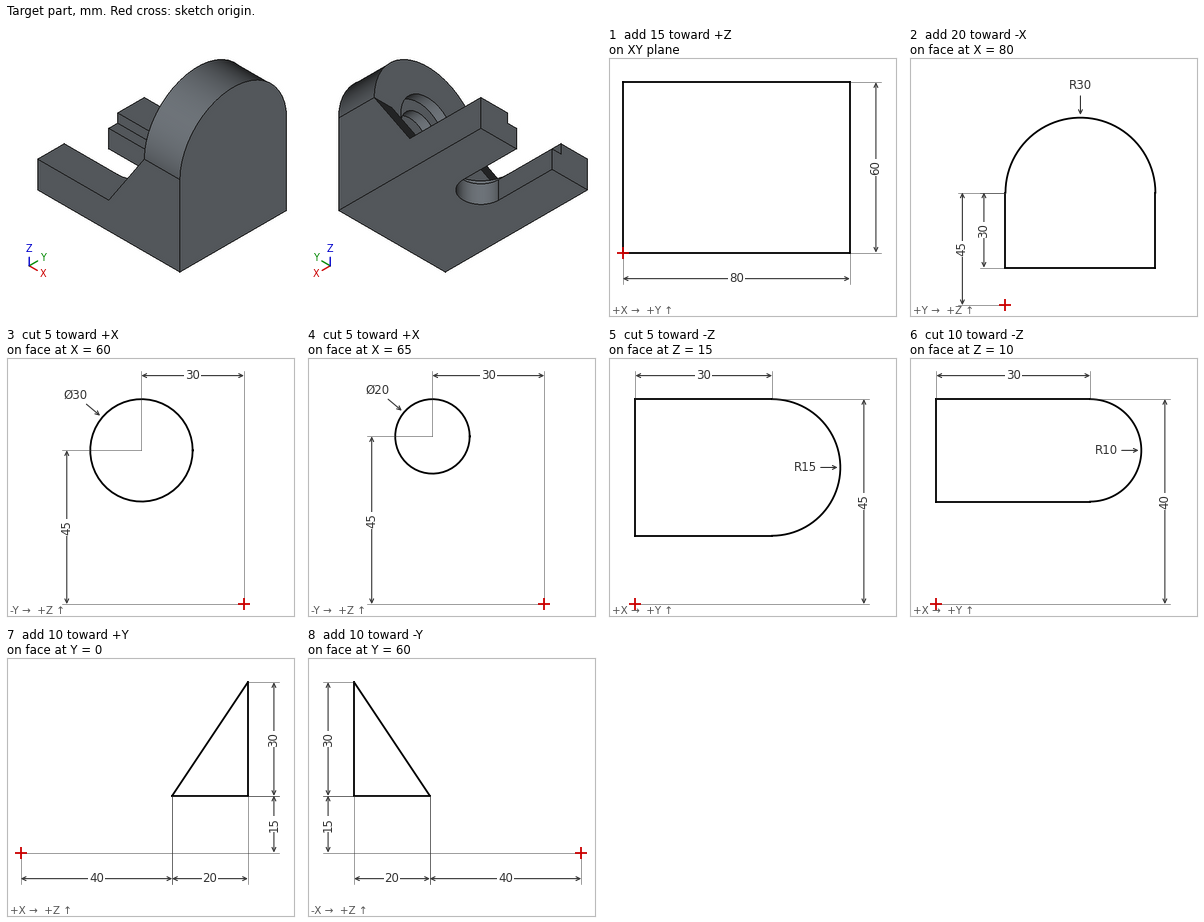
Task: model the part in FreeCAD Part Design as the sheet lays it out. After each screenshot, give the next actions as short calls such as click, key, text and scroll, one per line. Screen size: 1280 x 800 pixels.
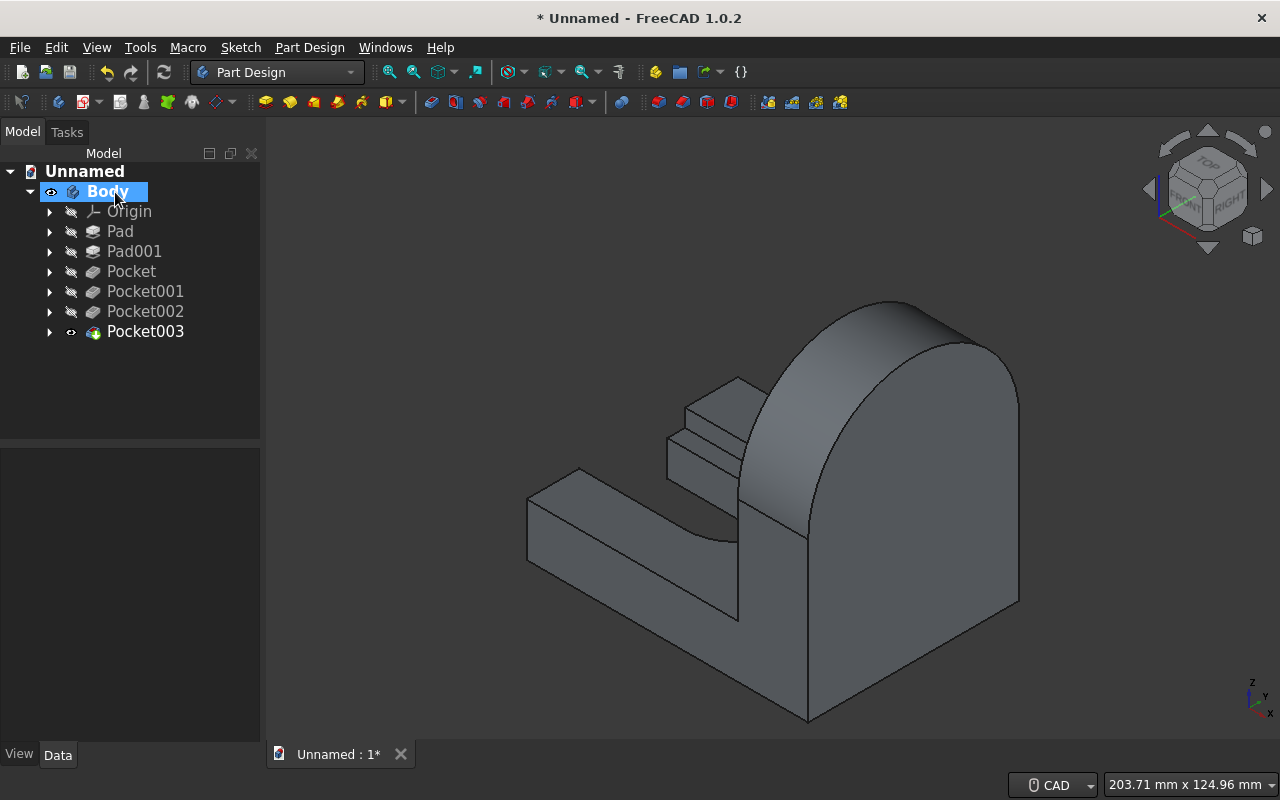
click(748, 647)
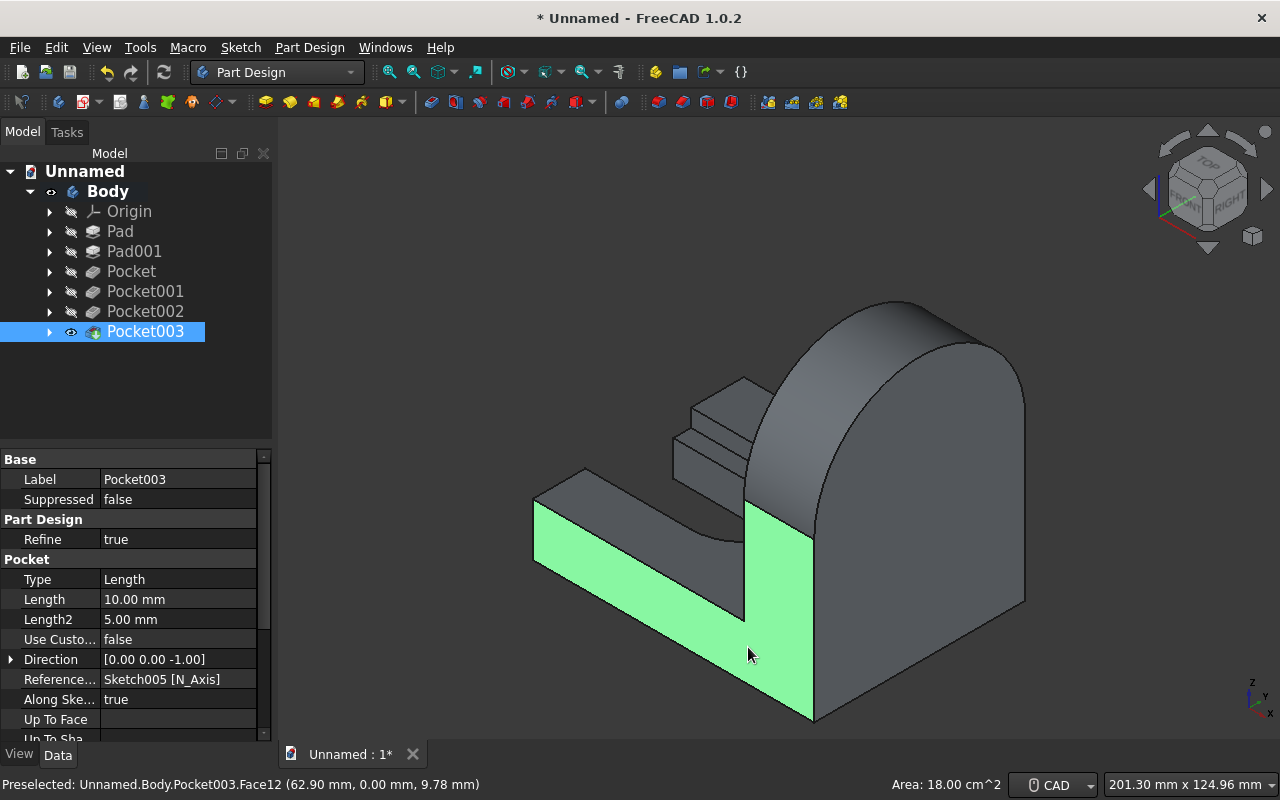
click(84, 102)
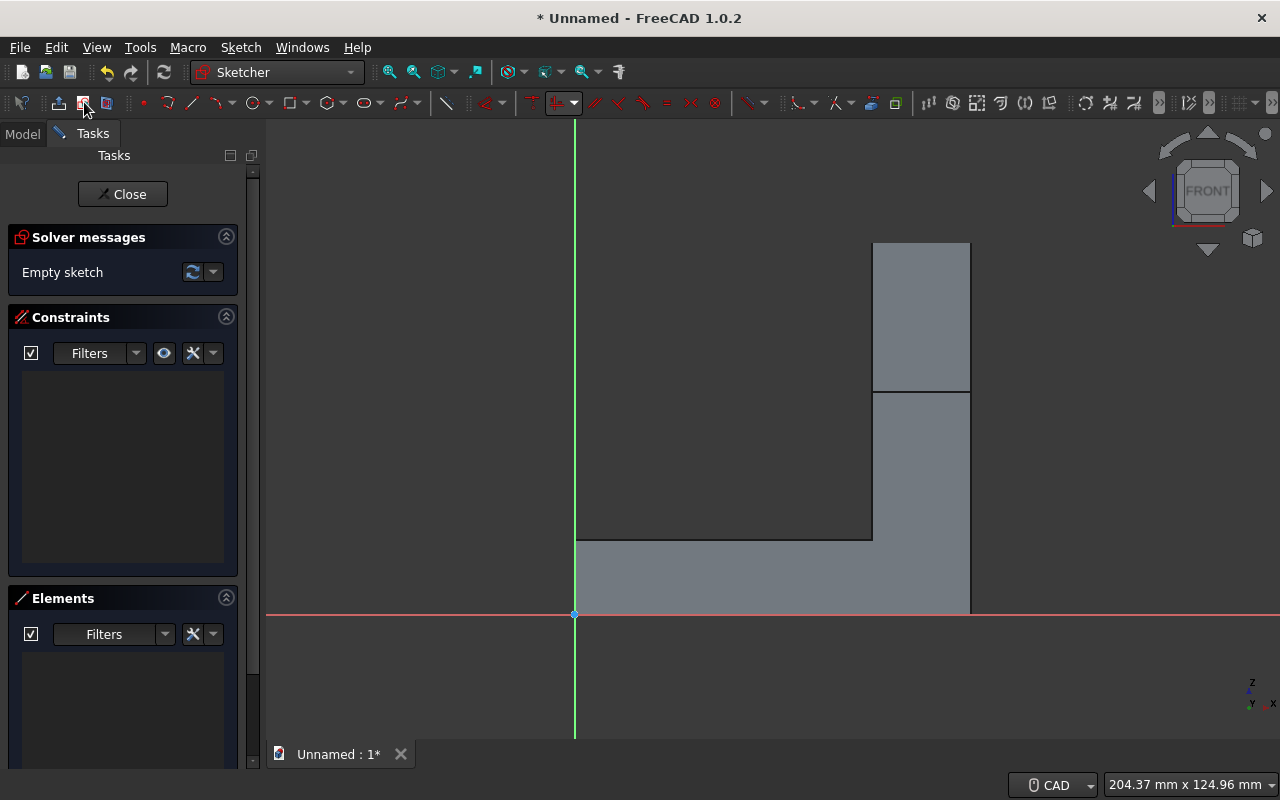
scroll(746, 594, up, 3)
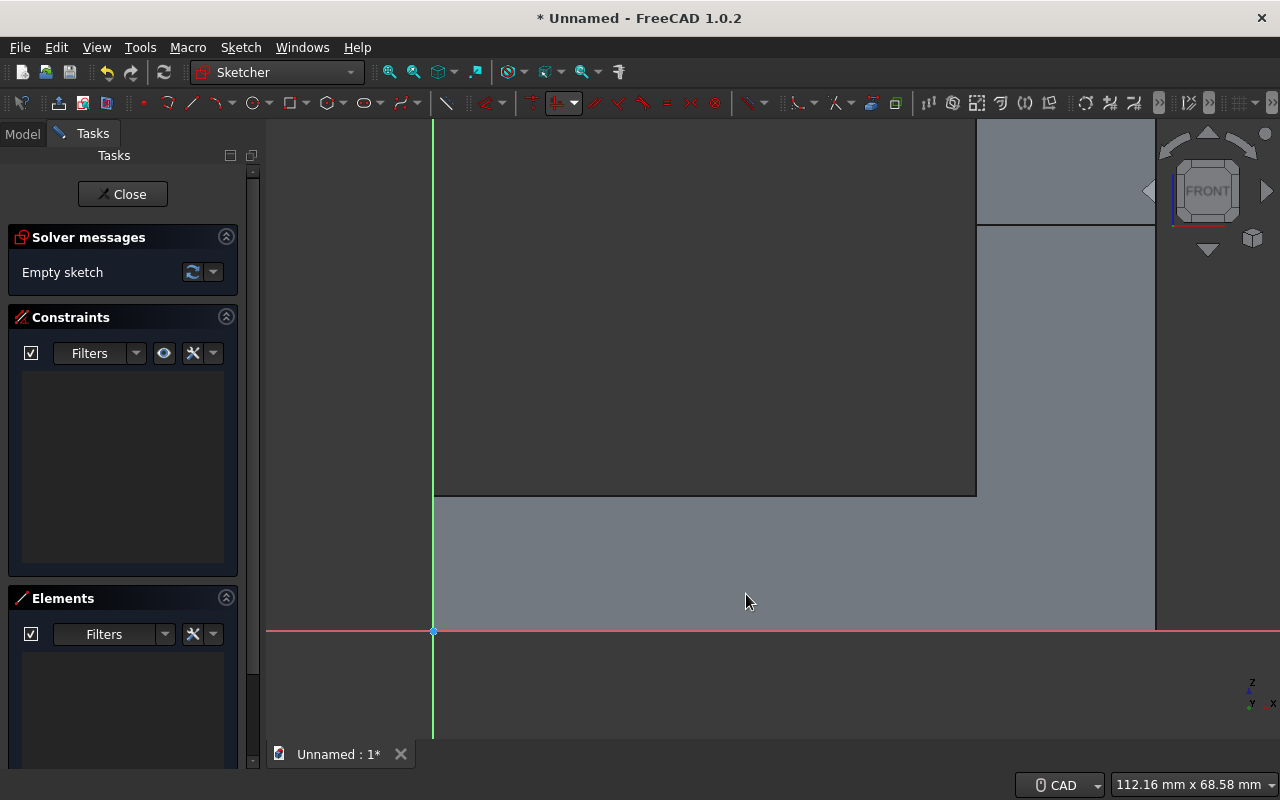
click(168, 104)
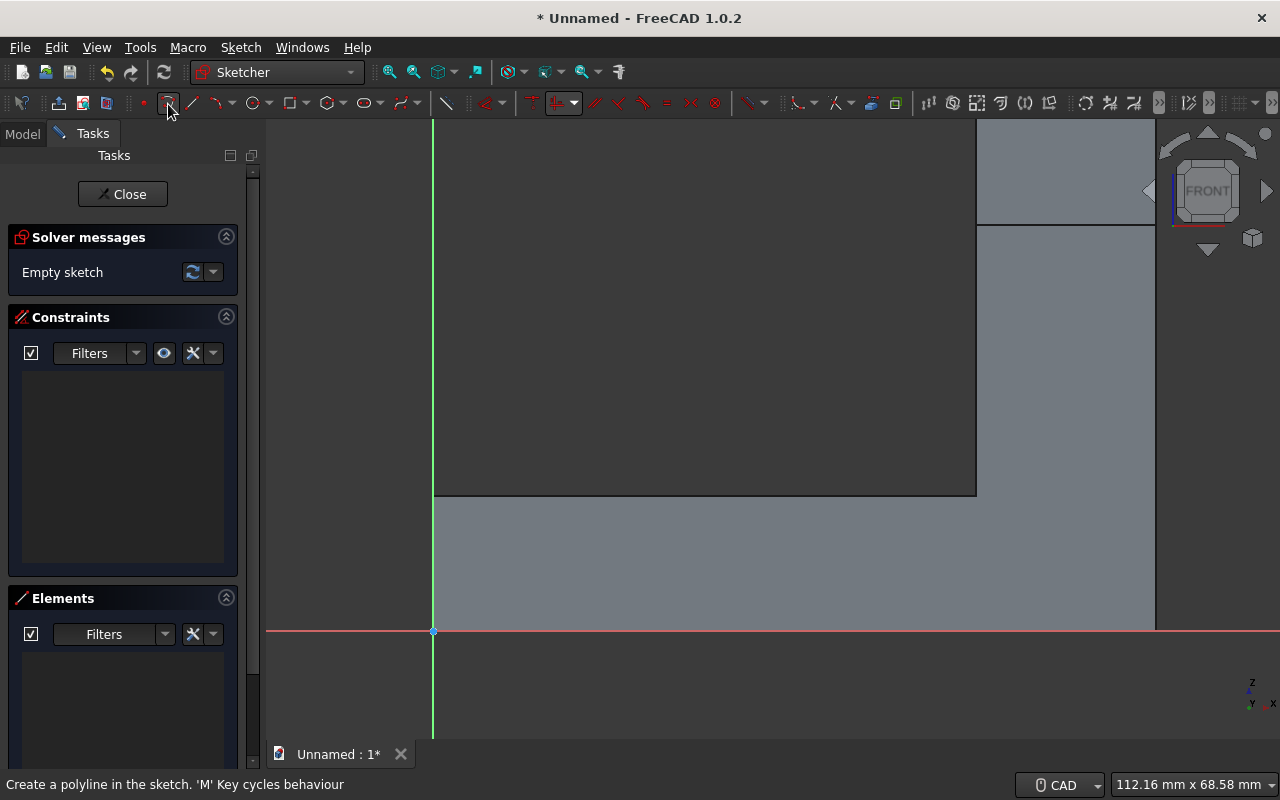
click(795, 496)
click(976, 496)
click(976, 225)
click(795, 497)
key(Escape)
key(Escape)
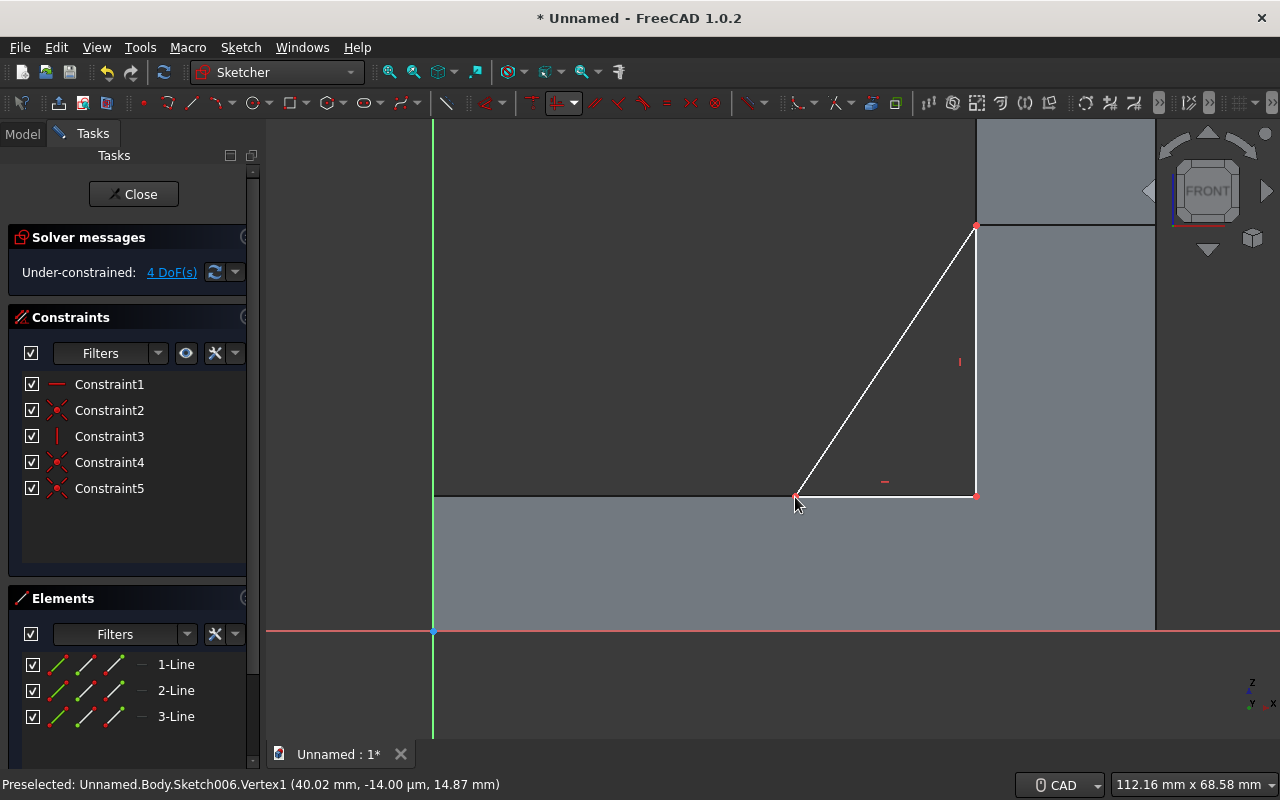
click(486, 104)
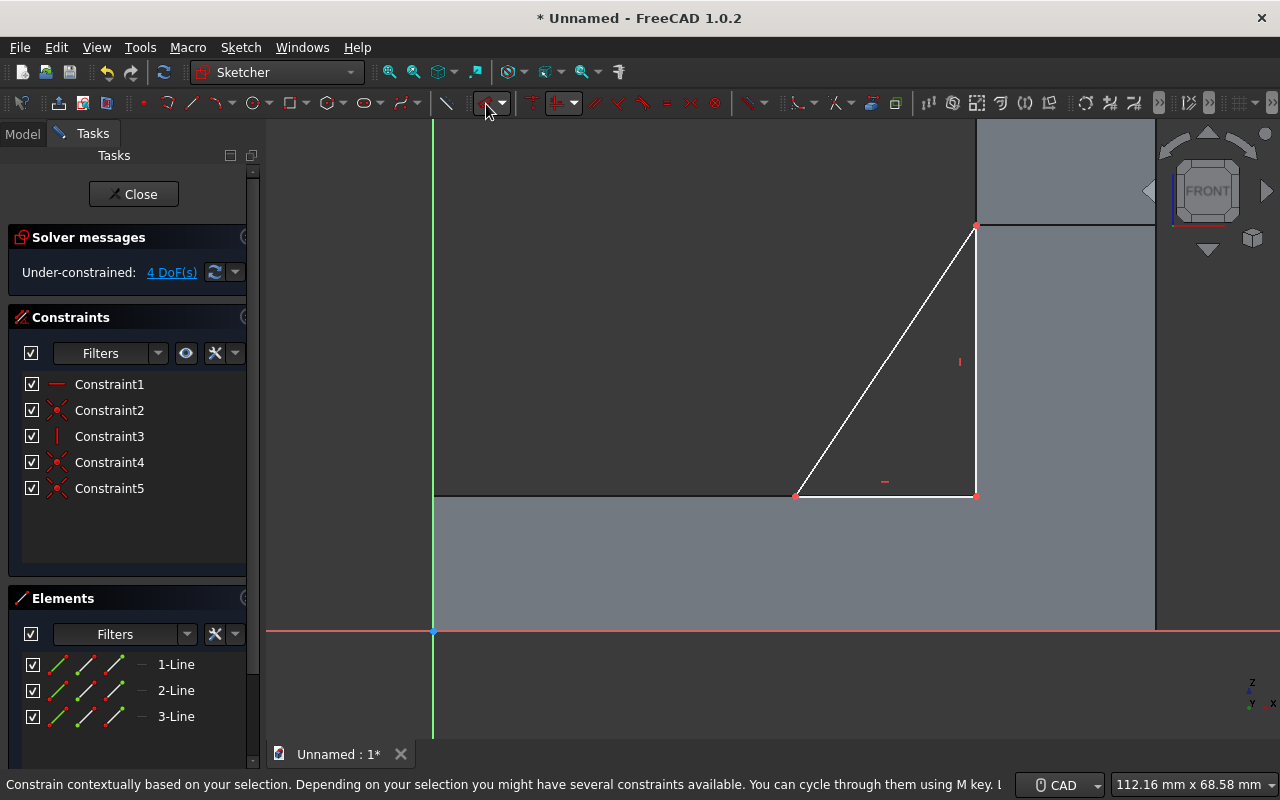
click(849, 497)
click(885, 531)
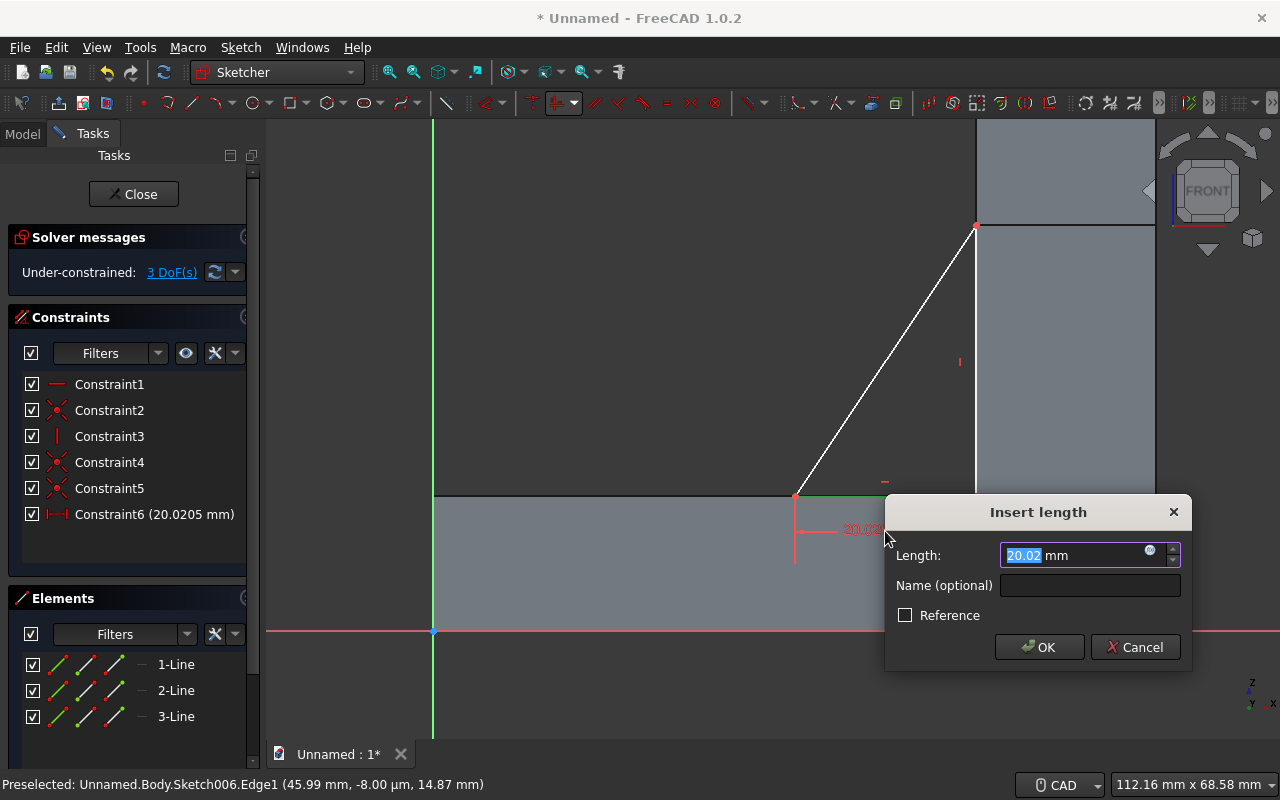
text(20)
key(Return)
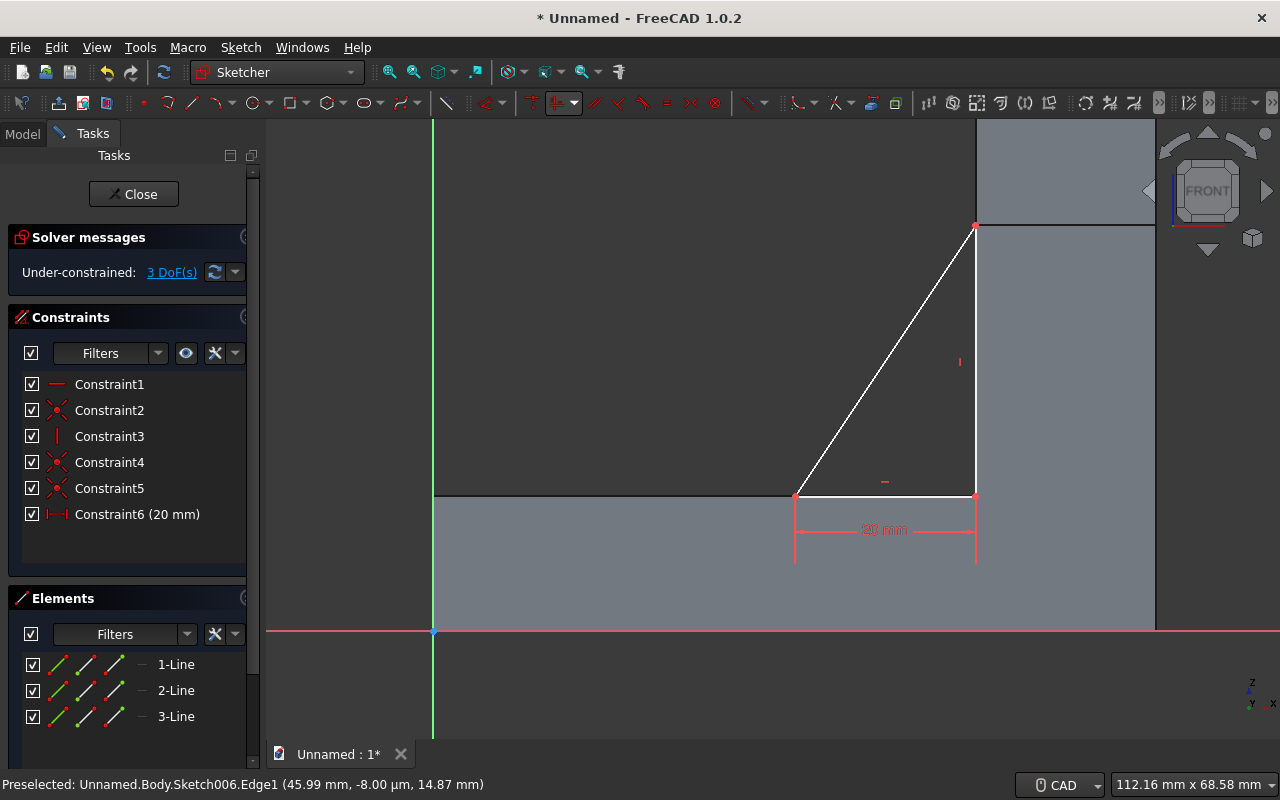
click(976, 416)
click(1010, 362)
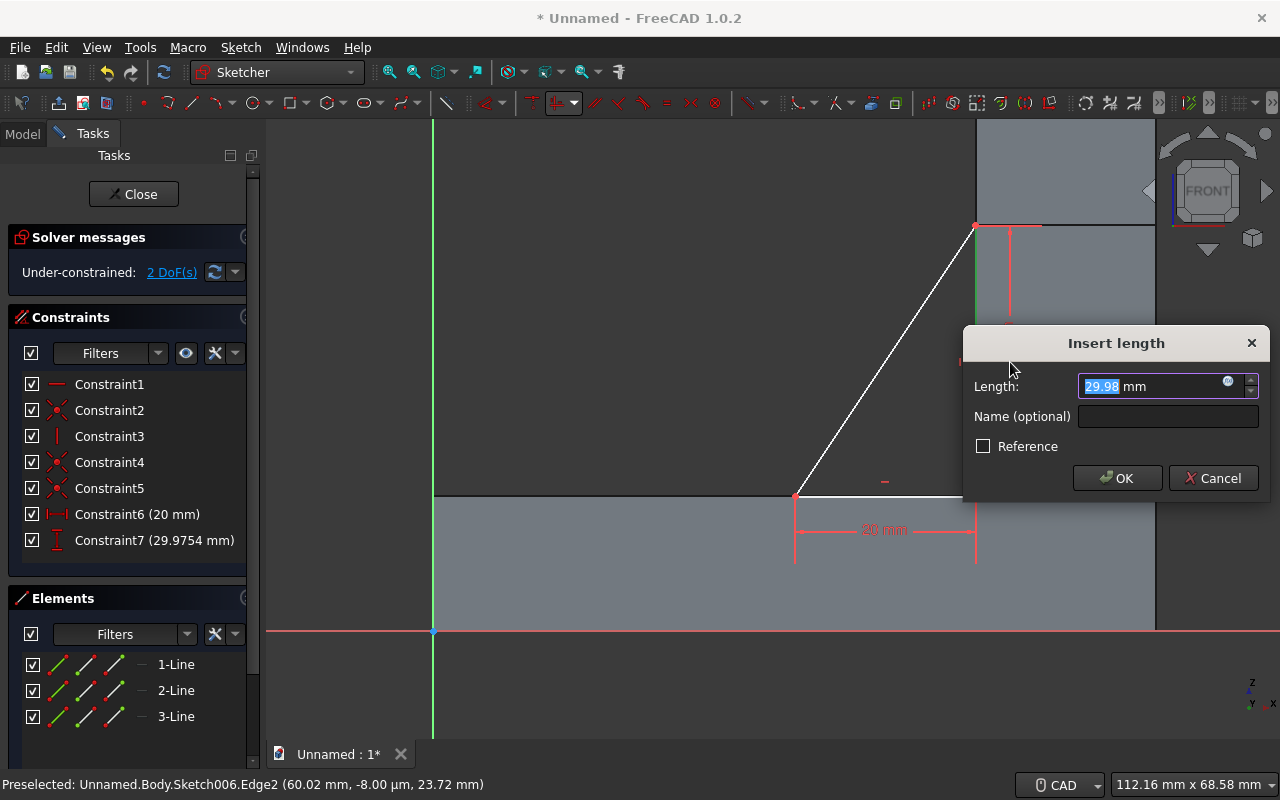
text(30)
key(Return)